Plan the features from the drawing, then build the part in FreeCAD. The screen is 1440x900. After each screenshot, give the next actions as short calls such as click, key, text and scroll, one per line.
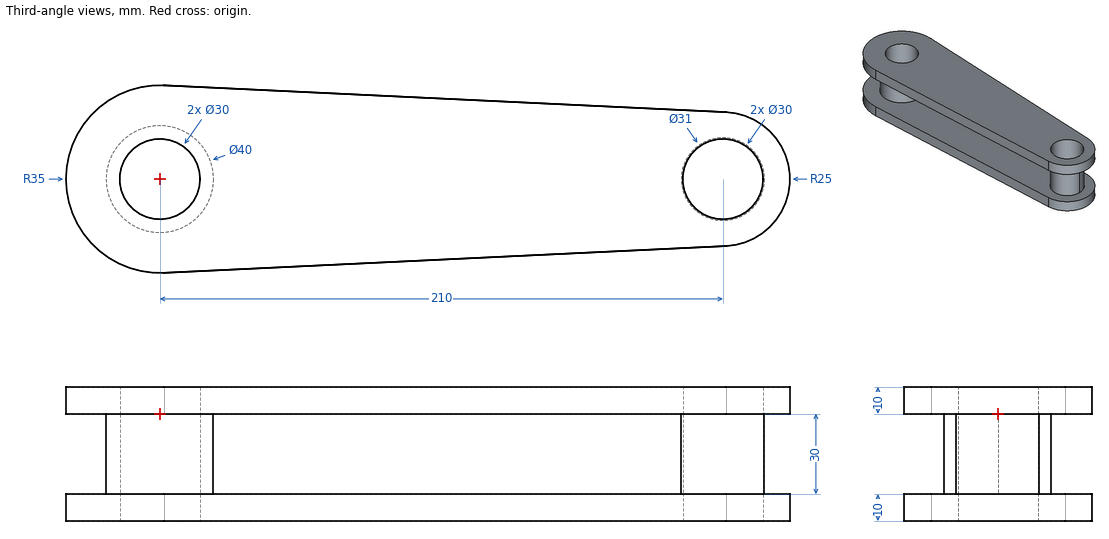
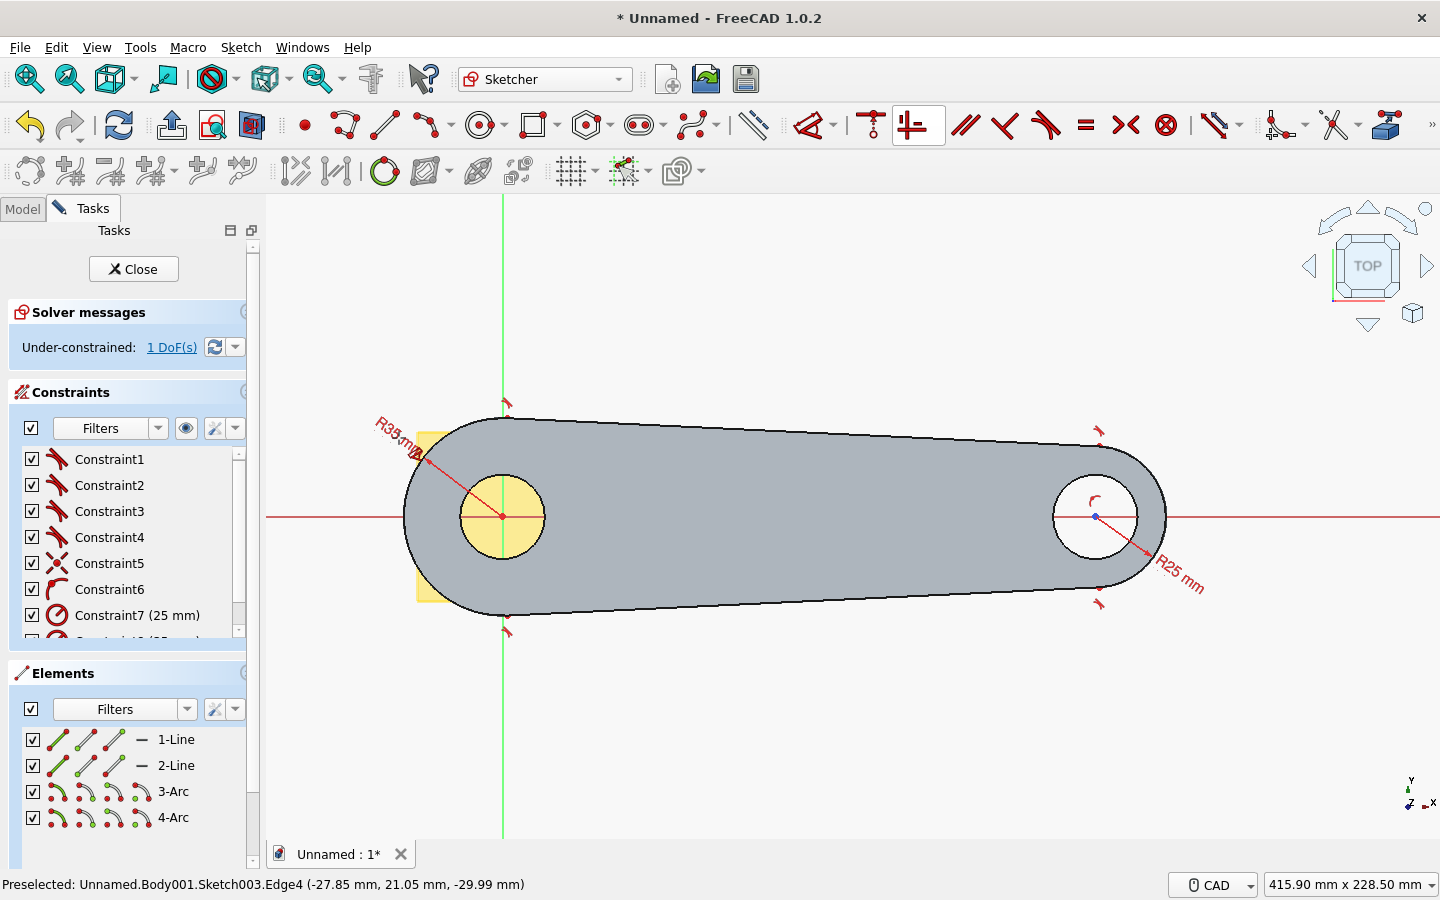
click(1096, 517)
click(799, 551)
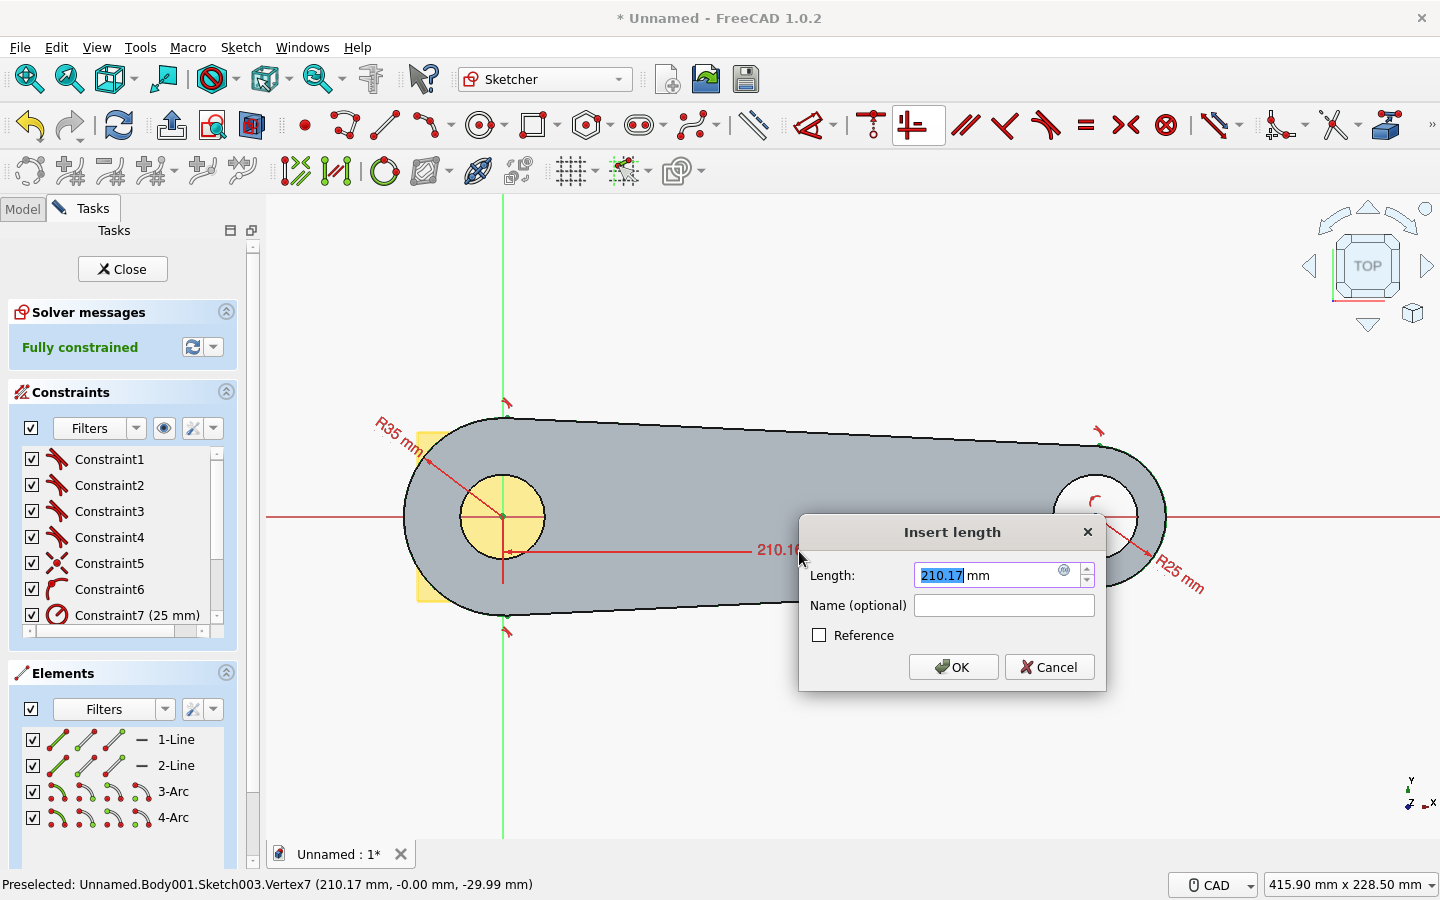
text(210)
key(Return)
key(Escape)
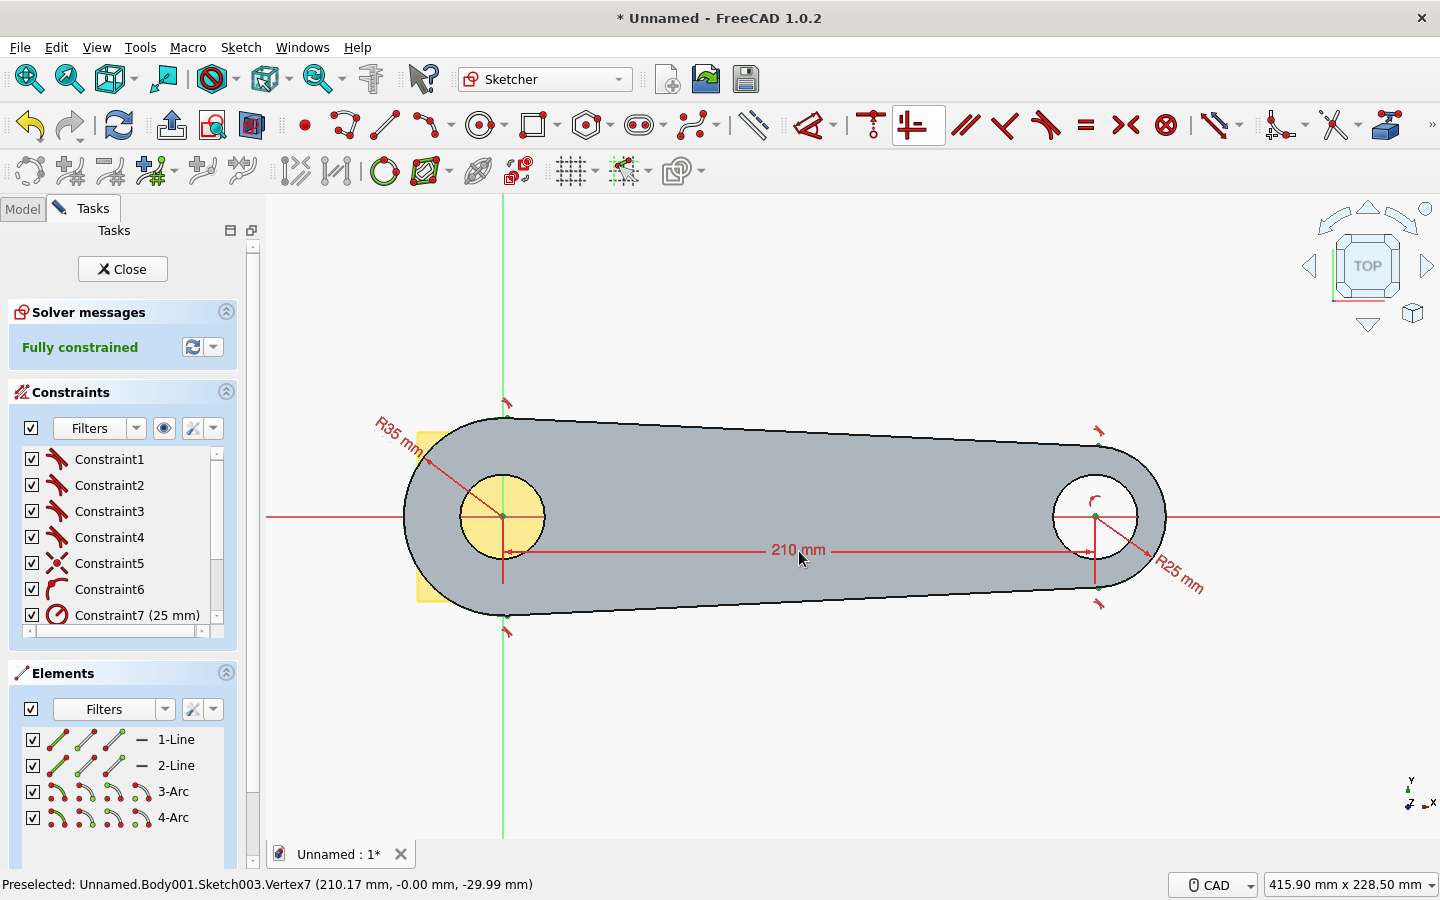
click(123, 269)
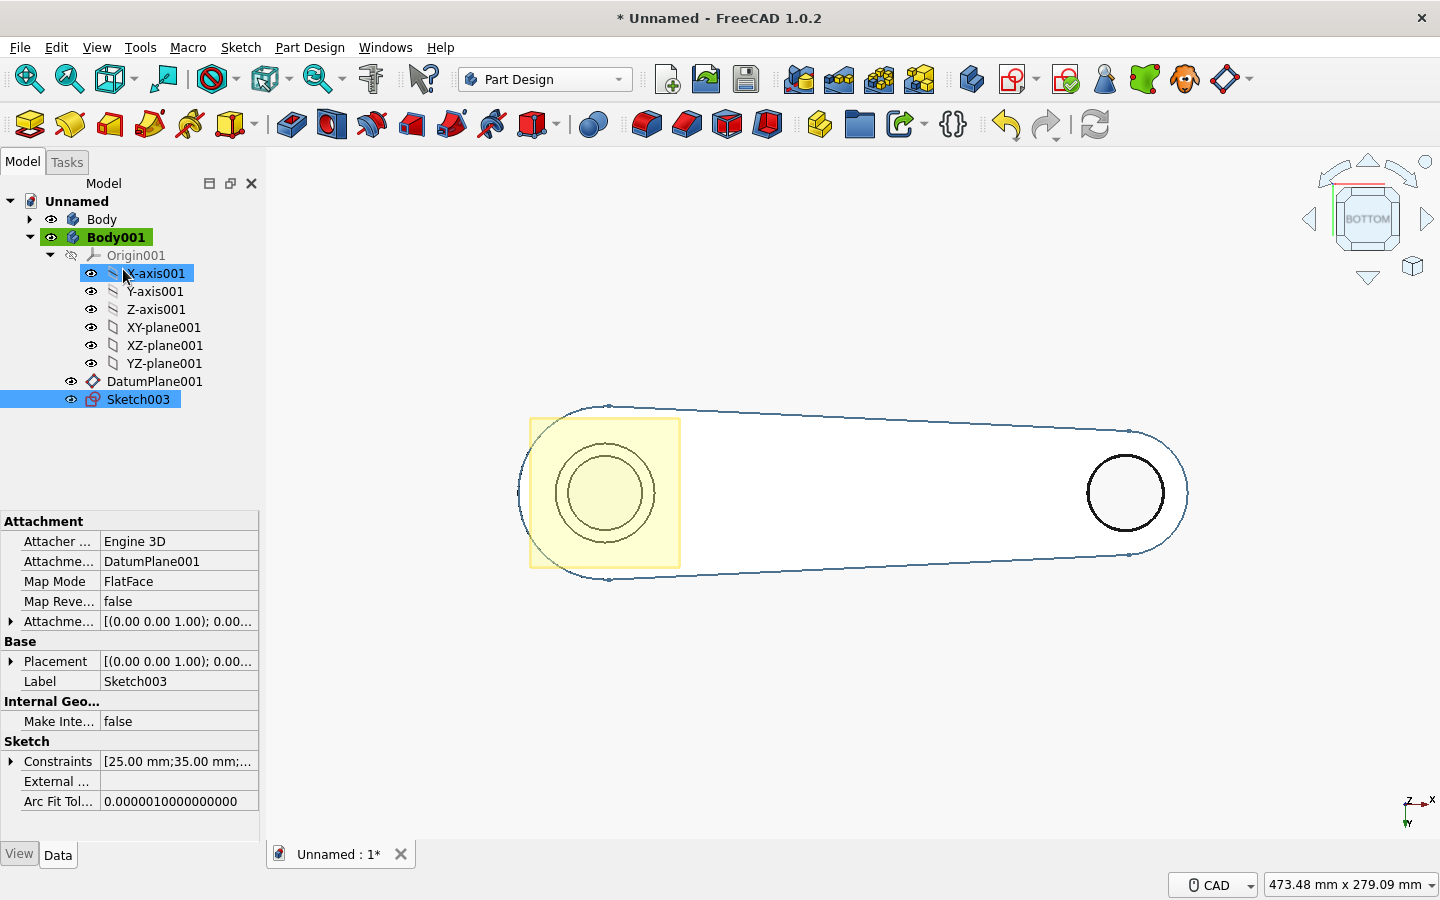
click(30, 124)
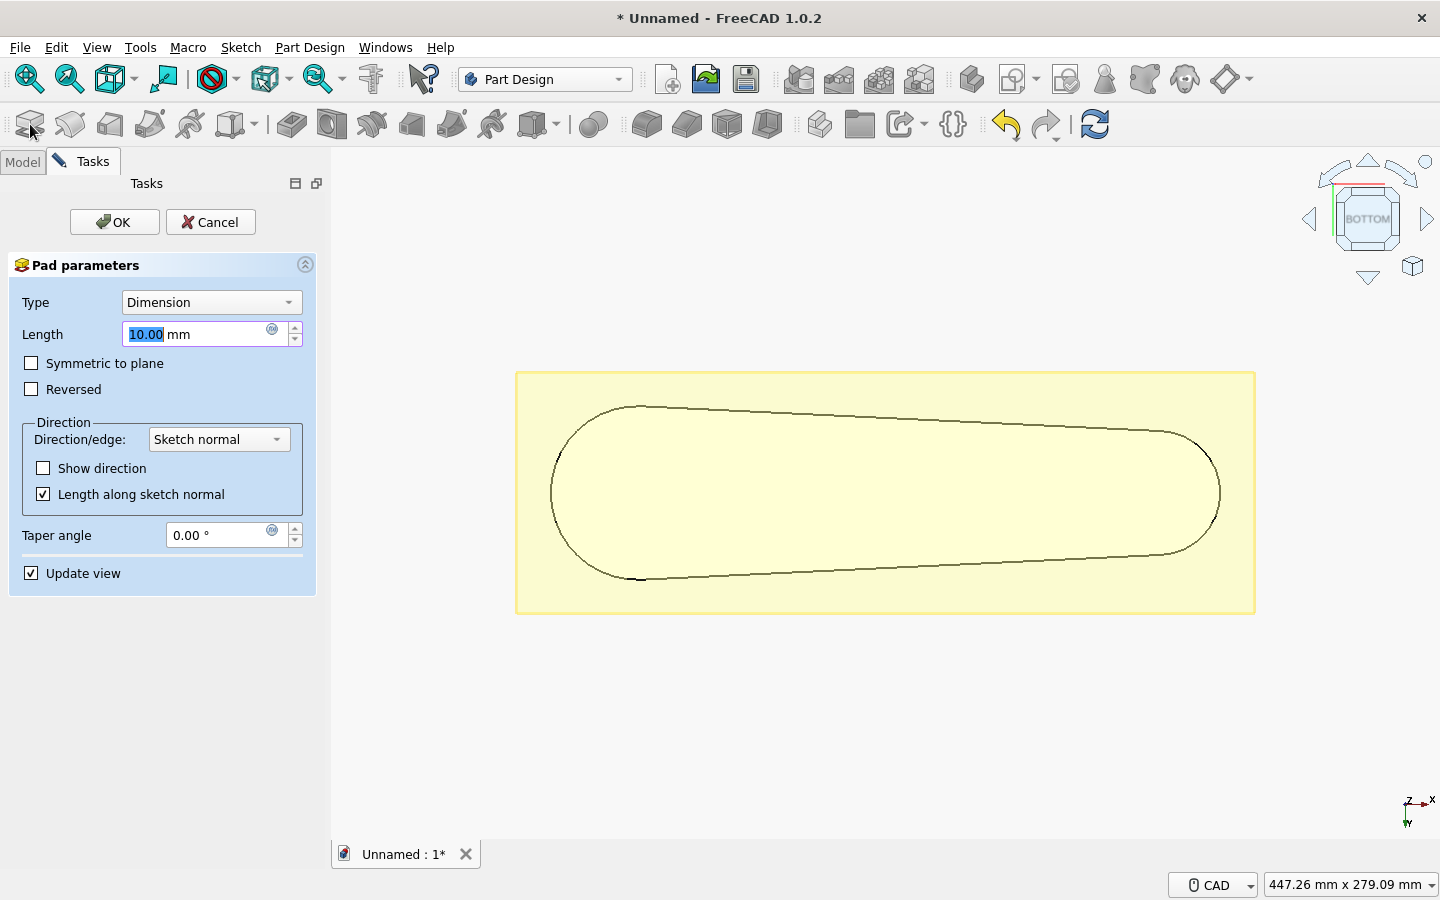
text(10)
key(Tab)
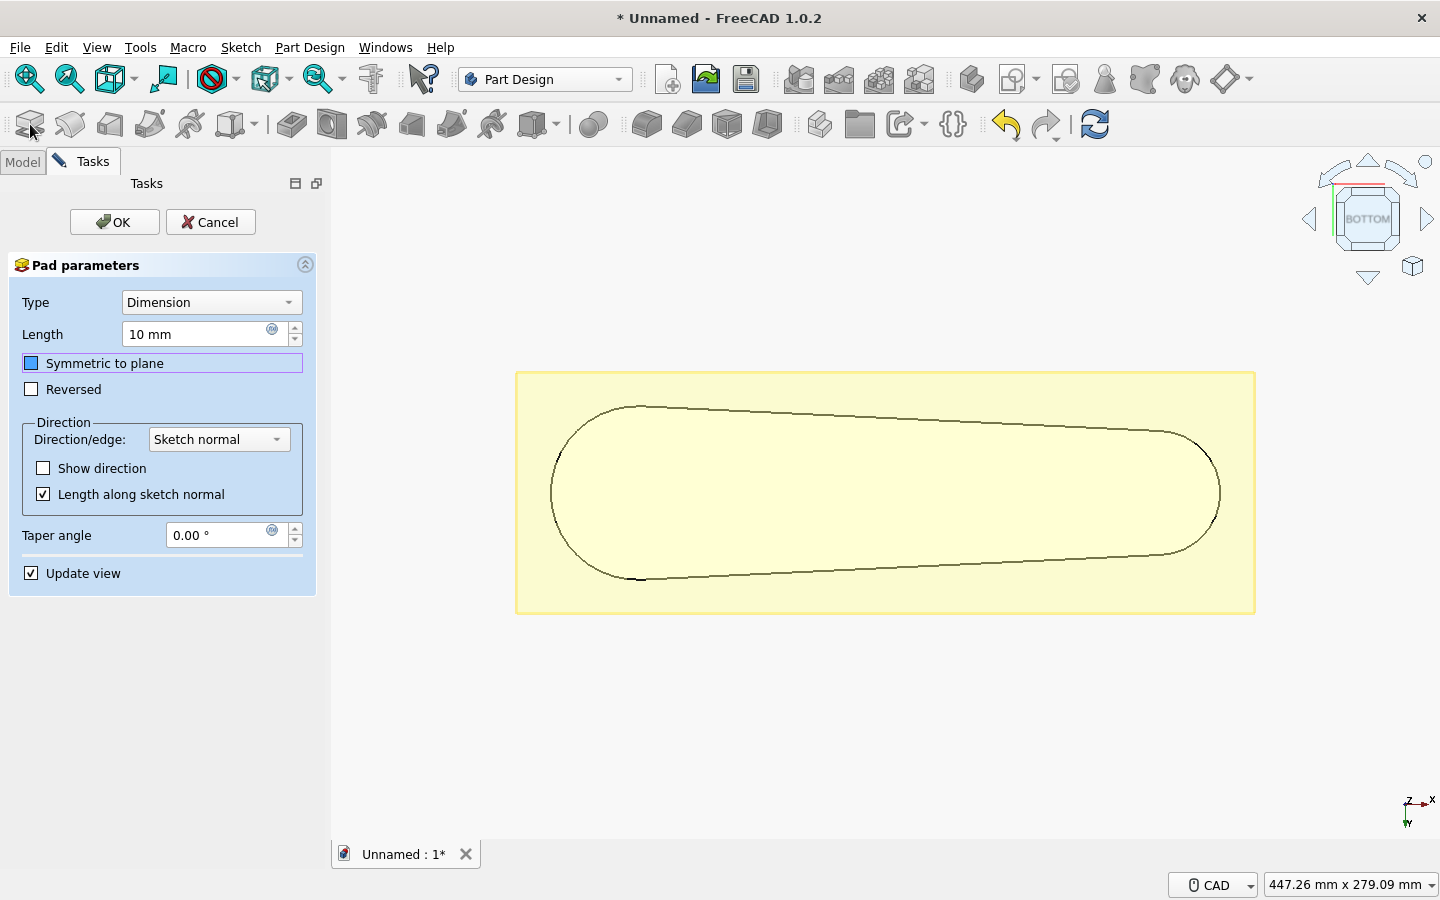
click(30, 389)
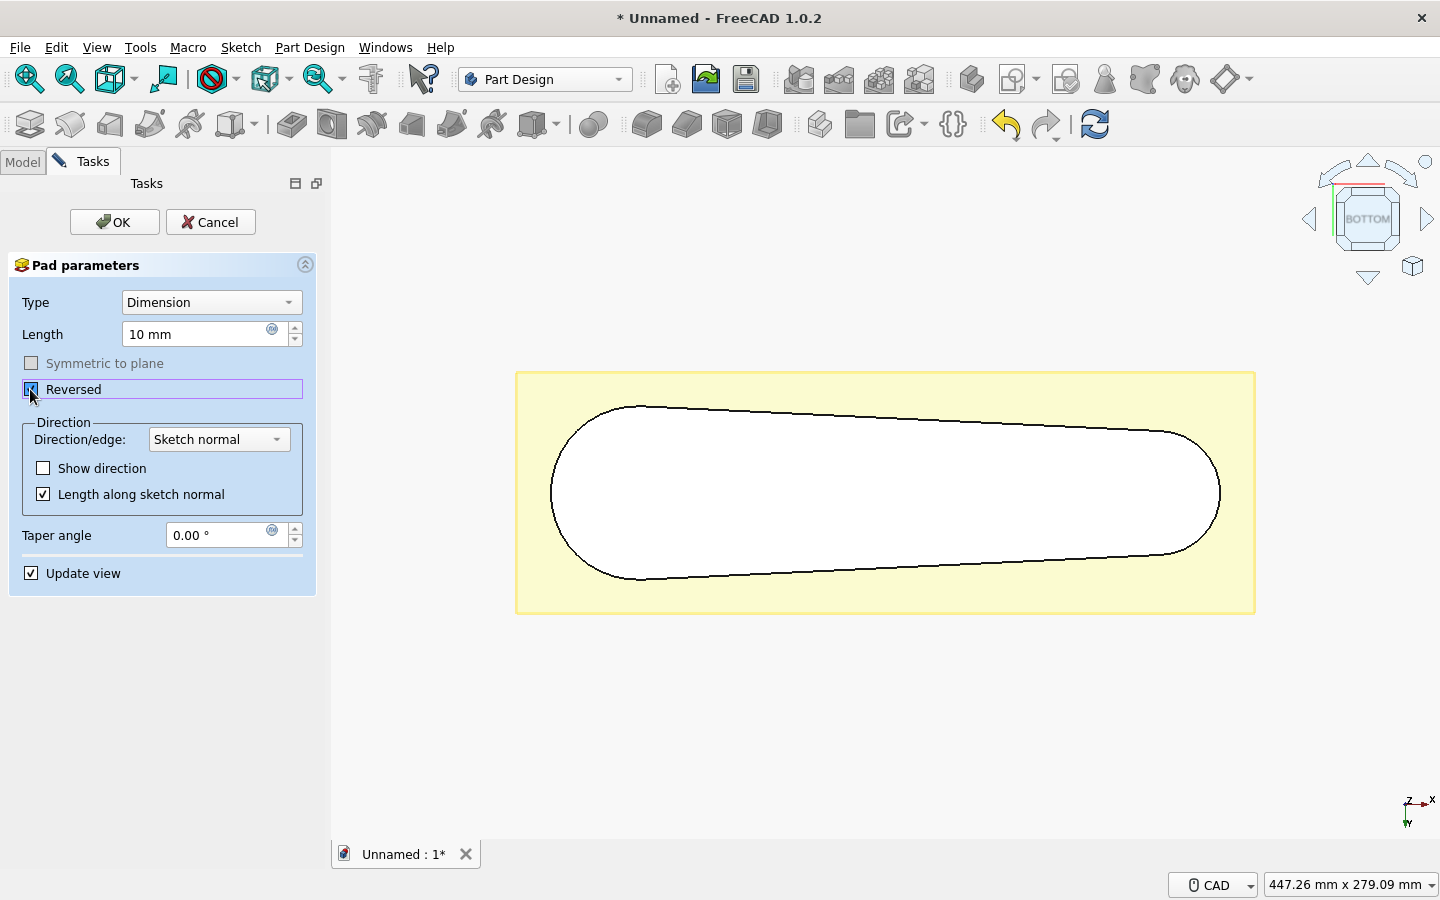
click(115, 222)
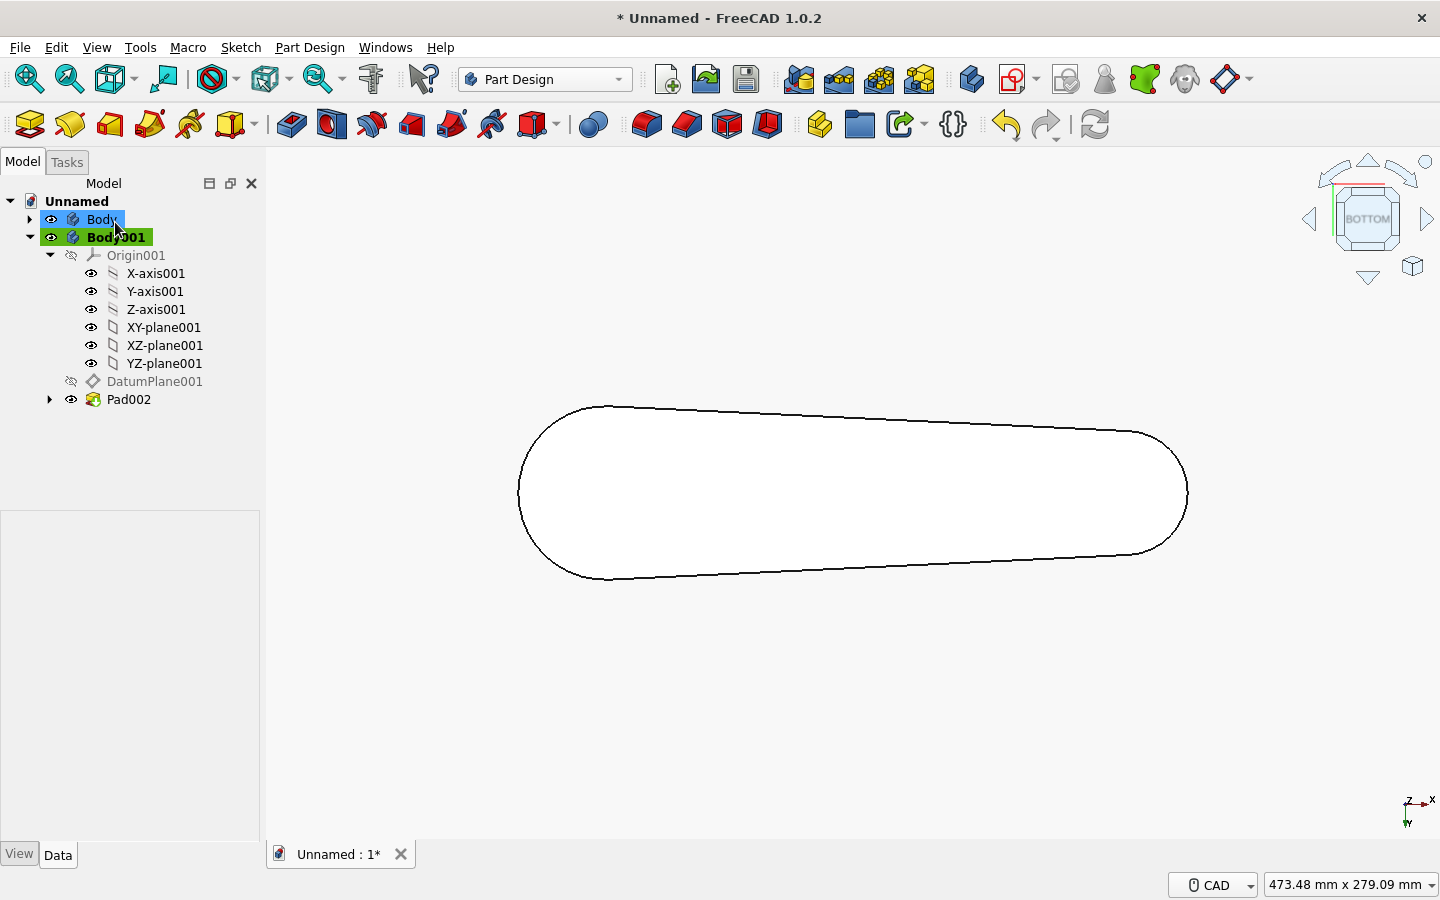
key(0)